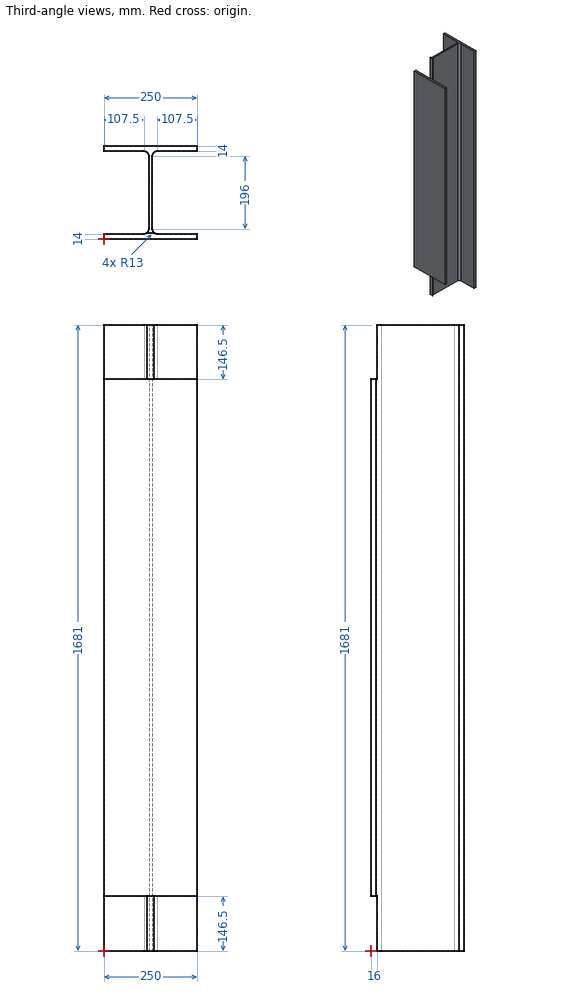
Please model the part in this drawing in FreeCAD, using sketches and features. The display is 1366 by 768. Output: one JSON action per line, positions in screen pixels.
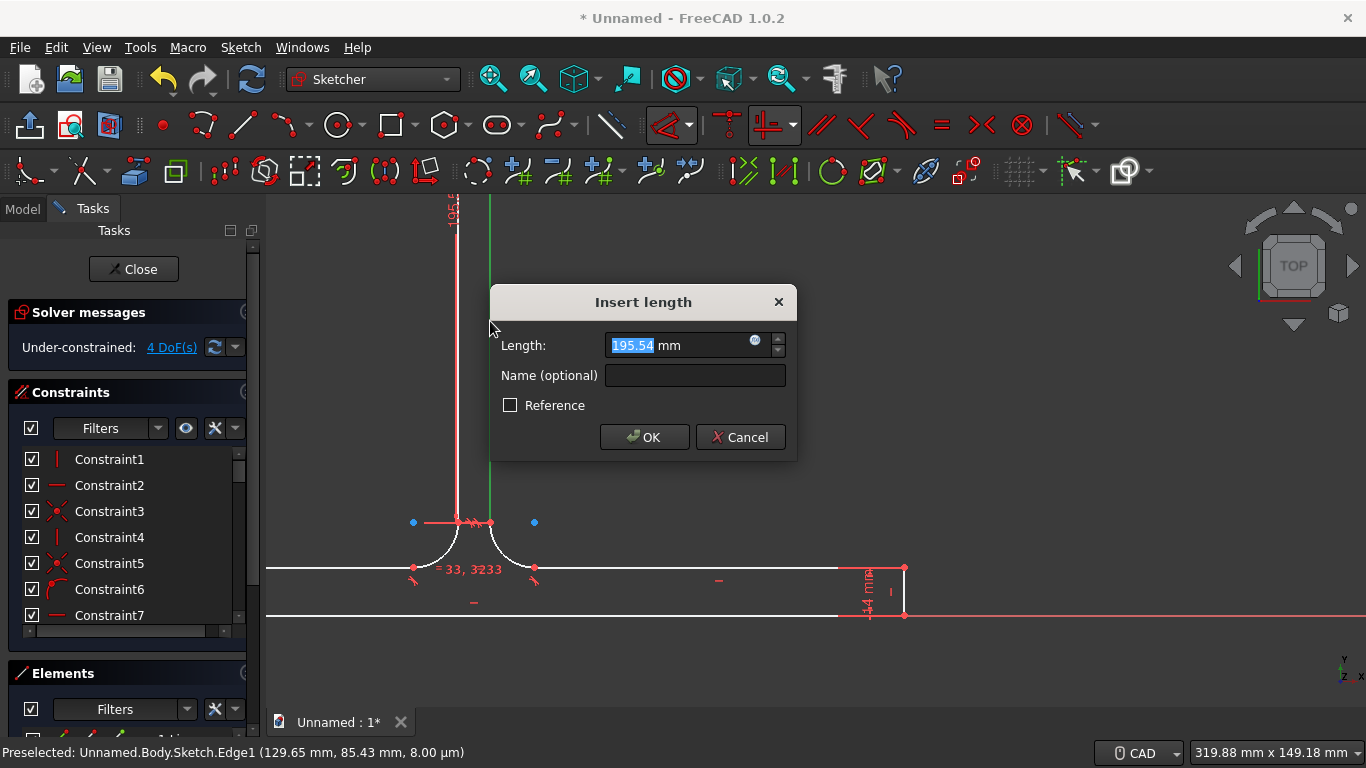
{"action": "type", "text": "196"}
{"action": "key", "text": "Return"}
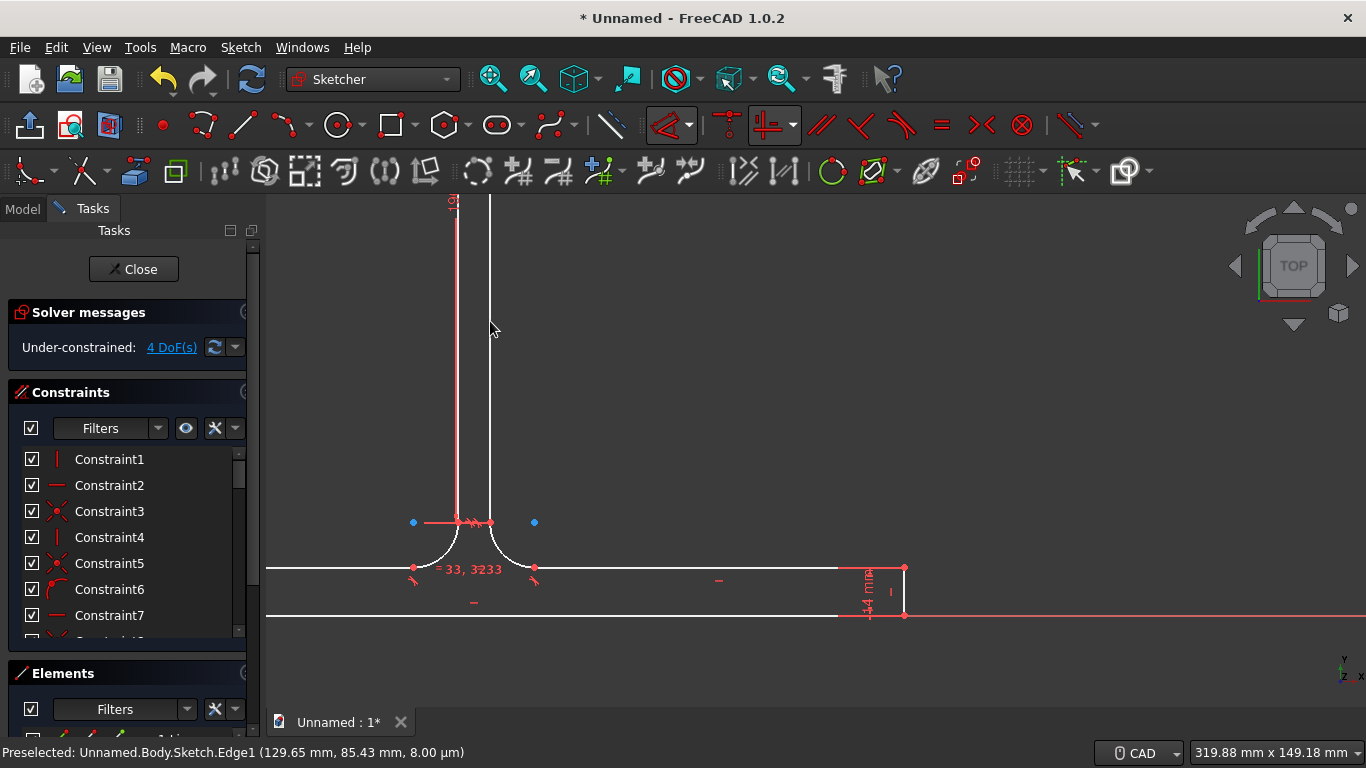
{"action": "scroll", "coordinate": [907, 604], "scroll_direction": "down", "scroll_amount": 5}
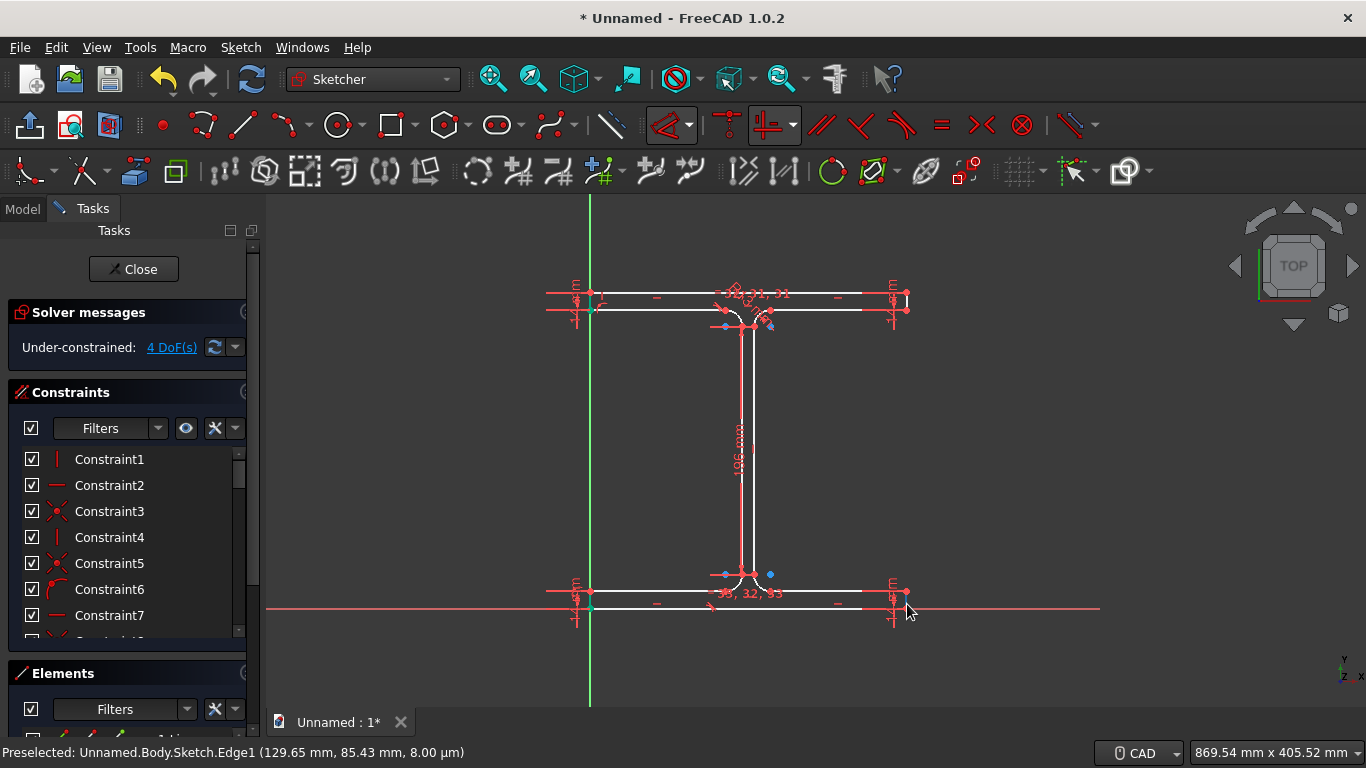
{"action": "left_click", "coordinate": [812, 293]}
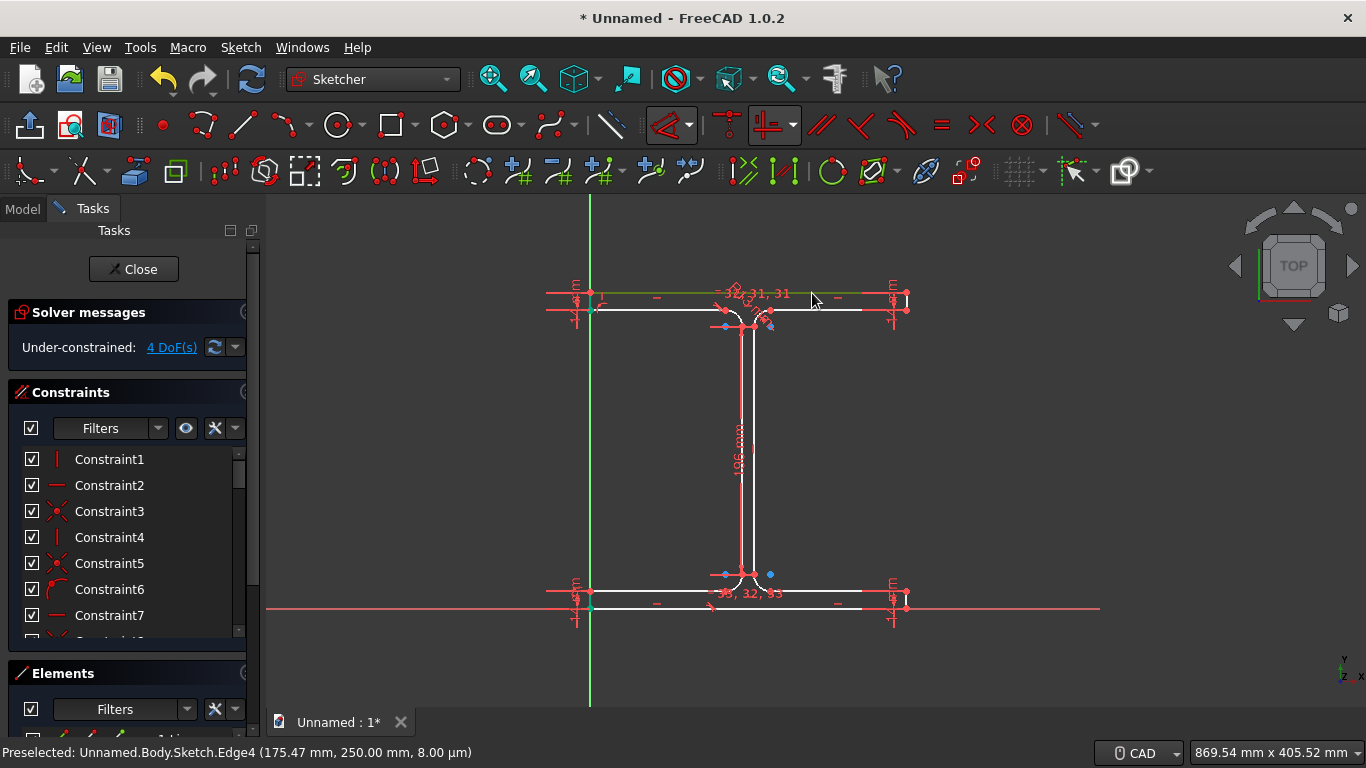
{"action": "left_click", "coordinate": [692, 126]}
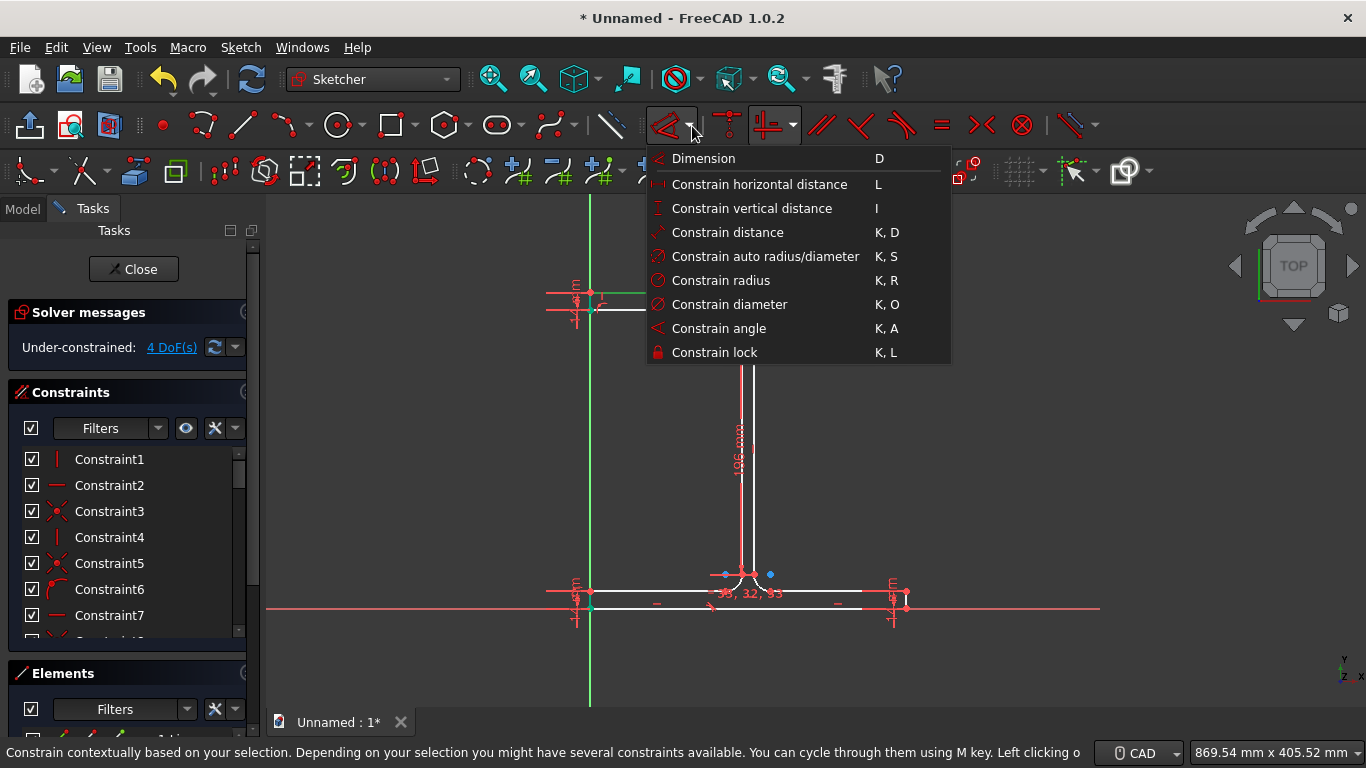
{"action": "left_click", "coordinate": [799, 184]}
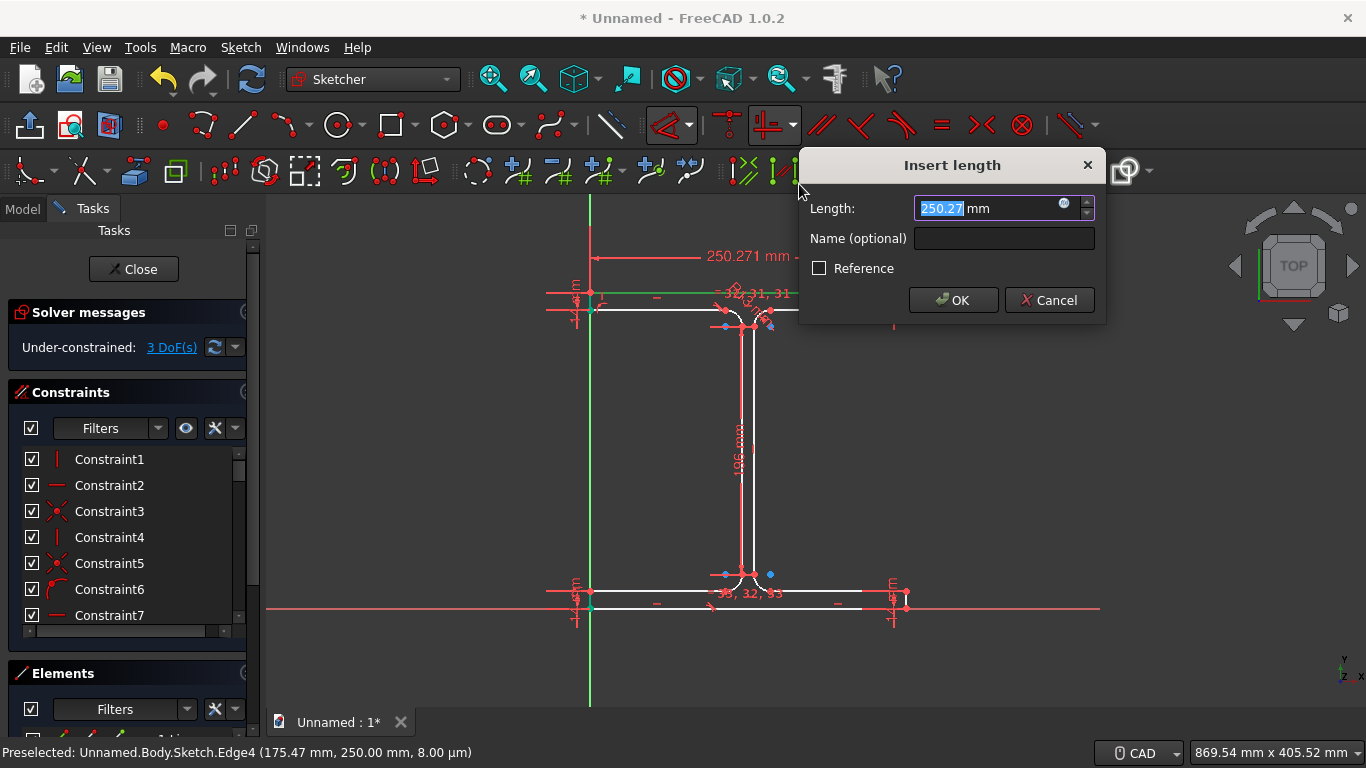
{"action": "type", "text": "250"}
{"action": "key", "text": "Return"}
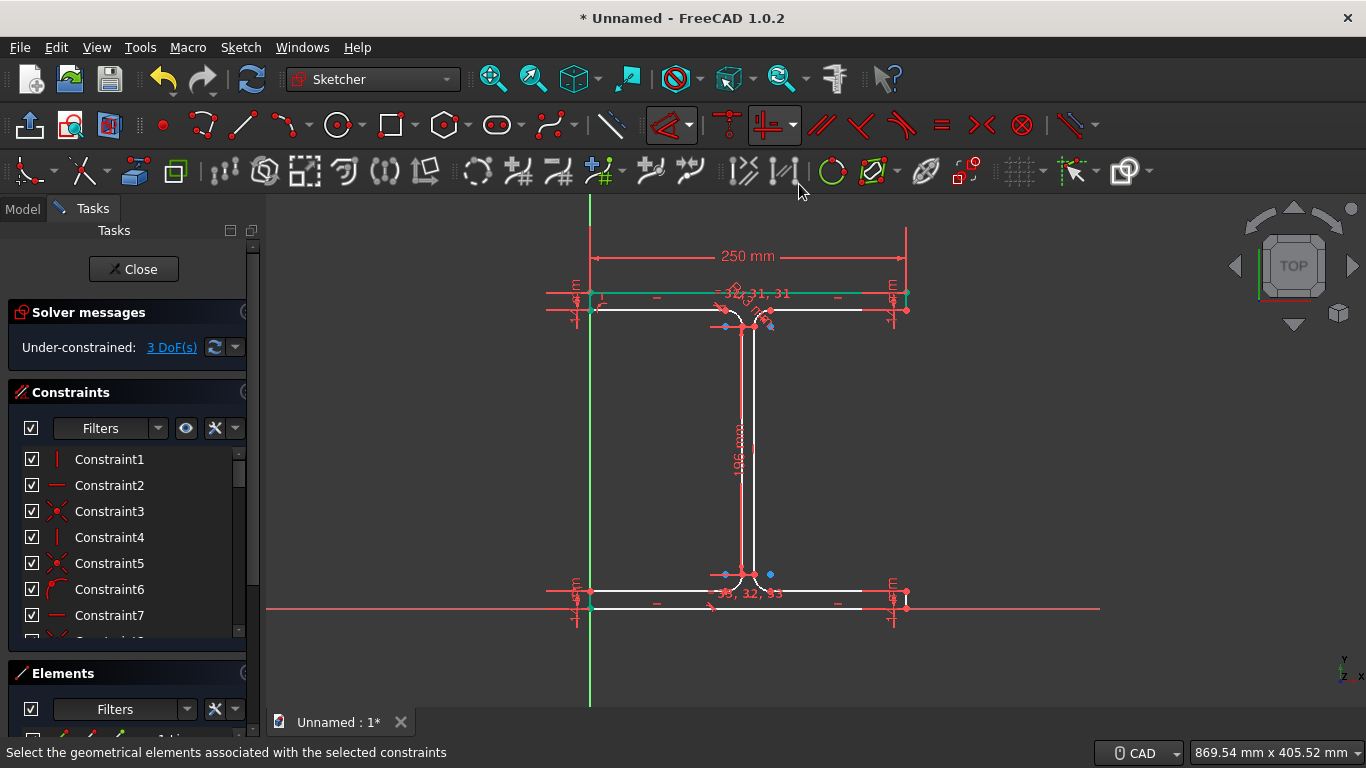
{"action": "left_click", "coordinate": [685, 609]}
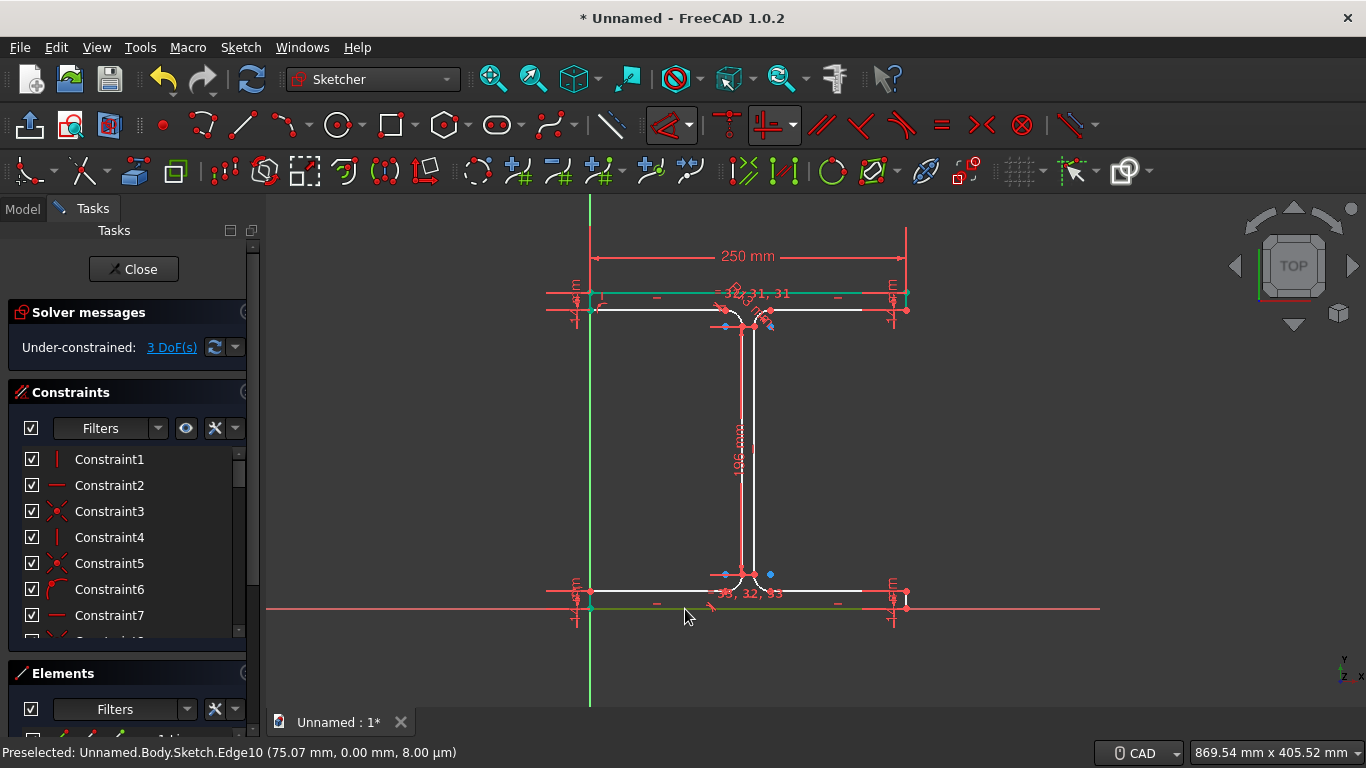
{"action": "key", "text": "l"}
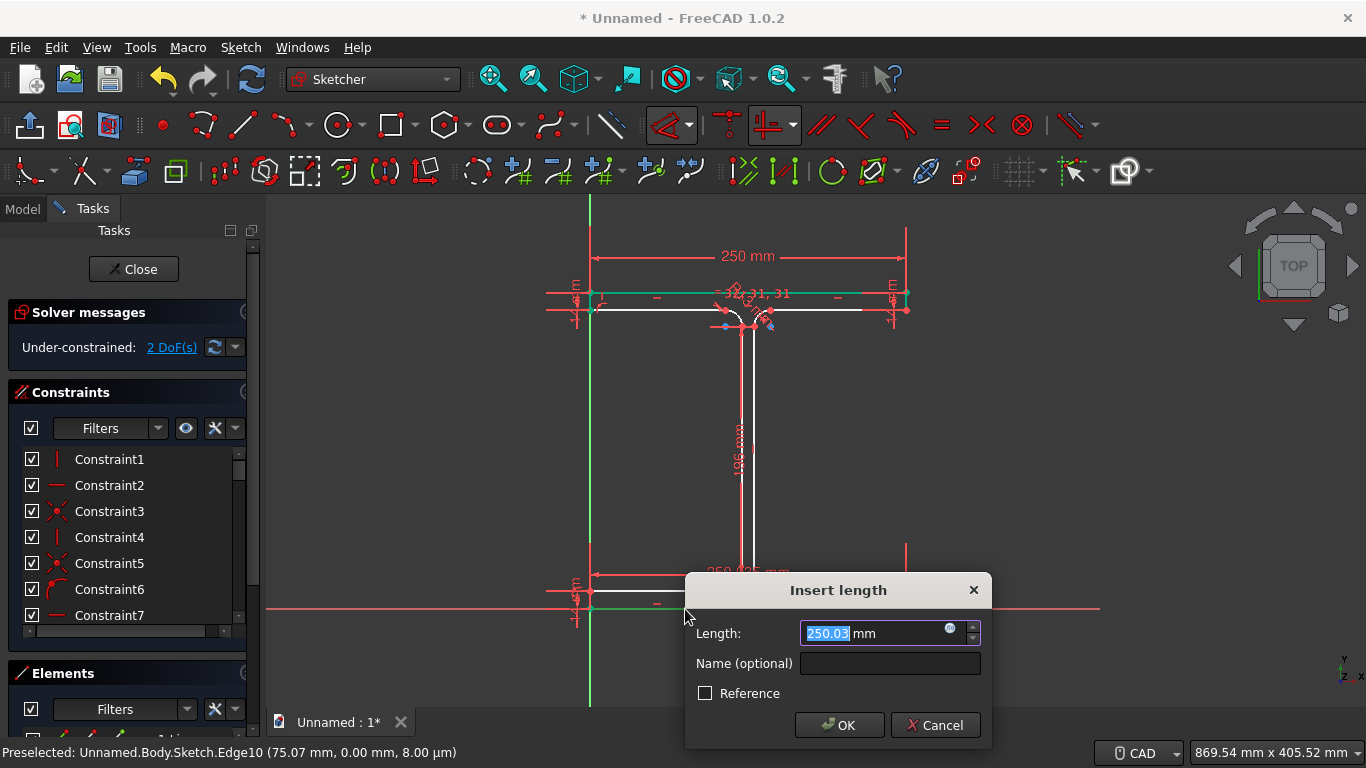
{"action": "type", "text": "250"}
{"action": "key", "text": "Return"}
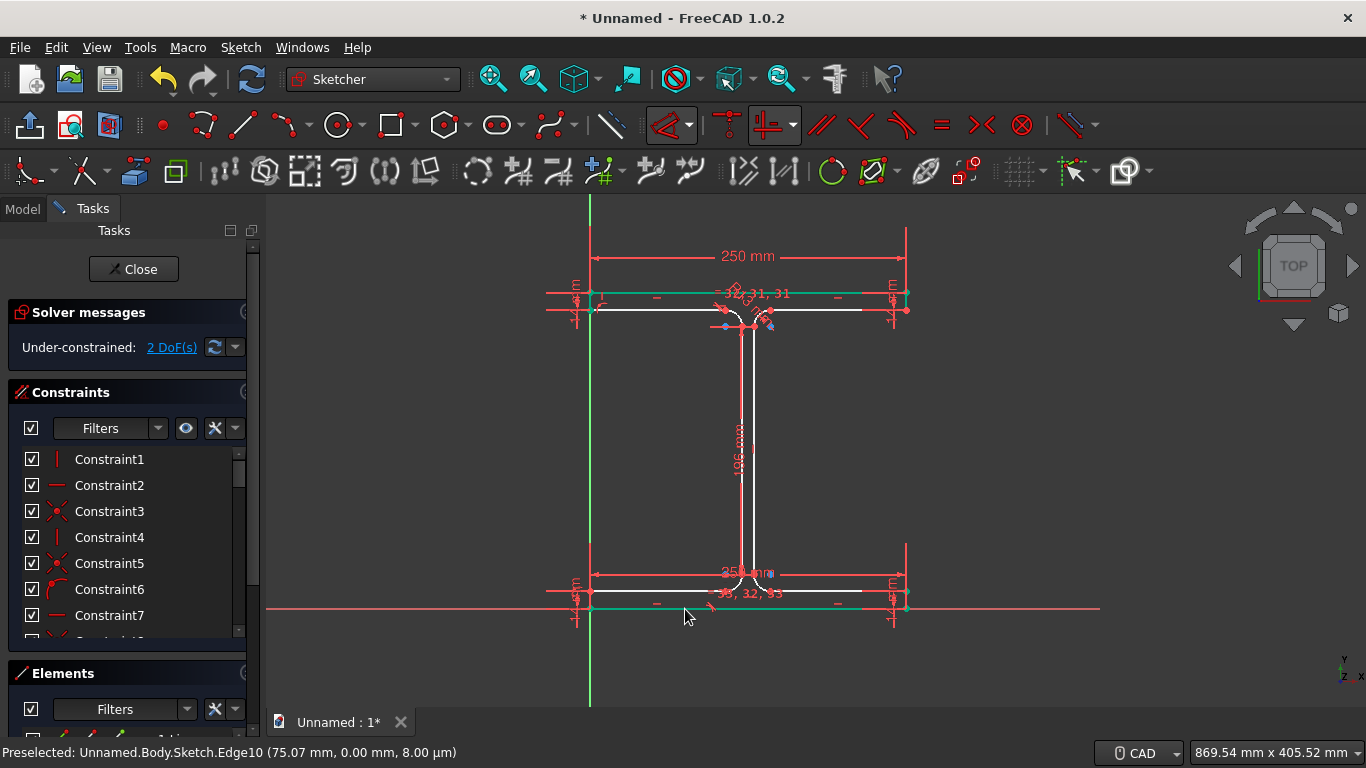
{"action": "left_click", "coordinate": [811, 310]}